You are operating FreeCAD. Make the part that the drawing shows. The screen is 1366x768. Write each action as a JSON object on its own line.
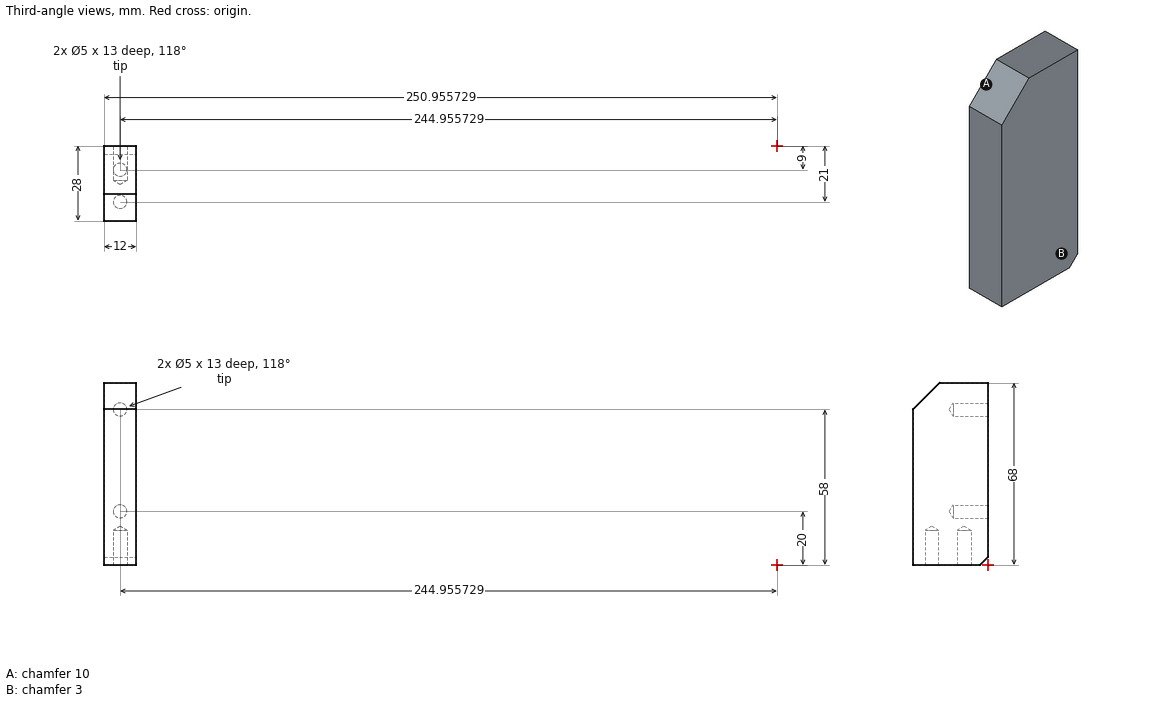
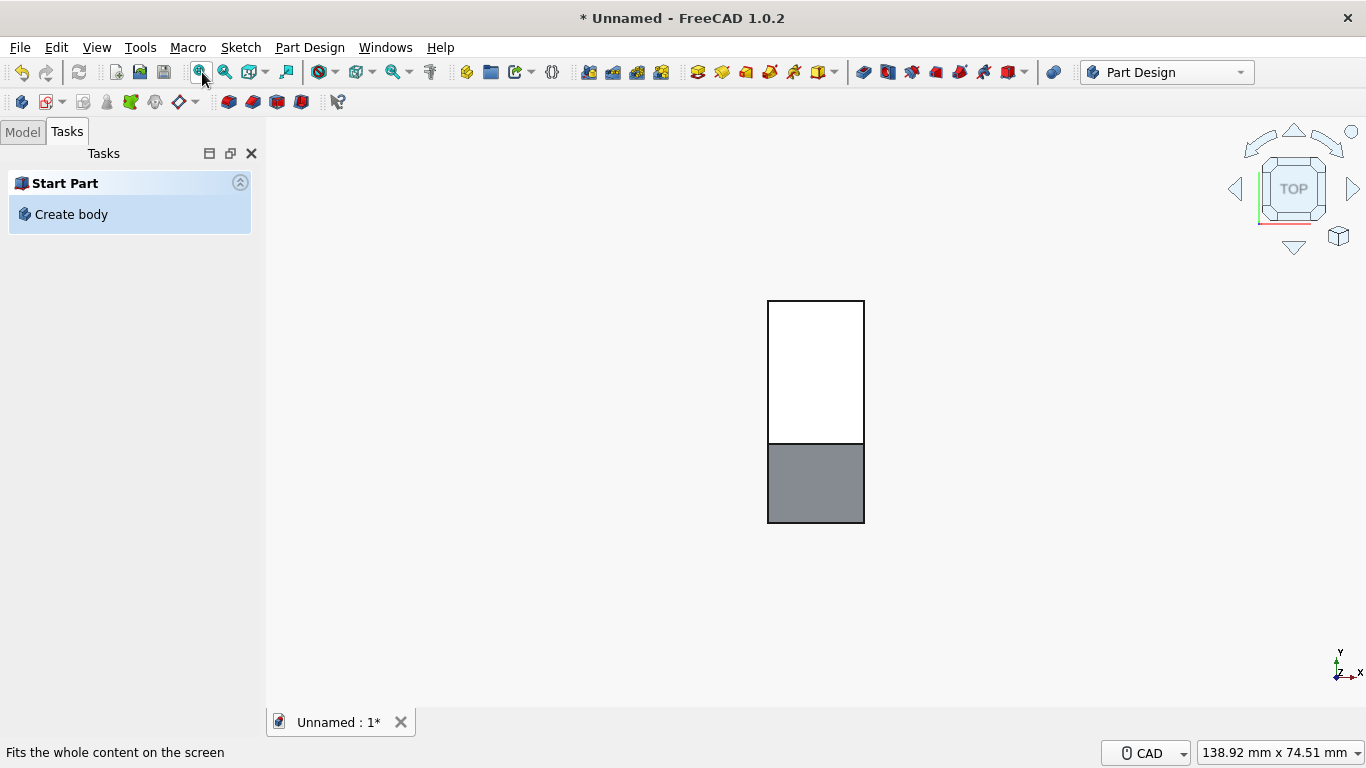
{"action": "key", "text": "1"}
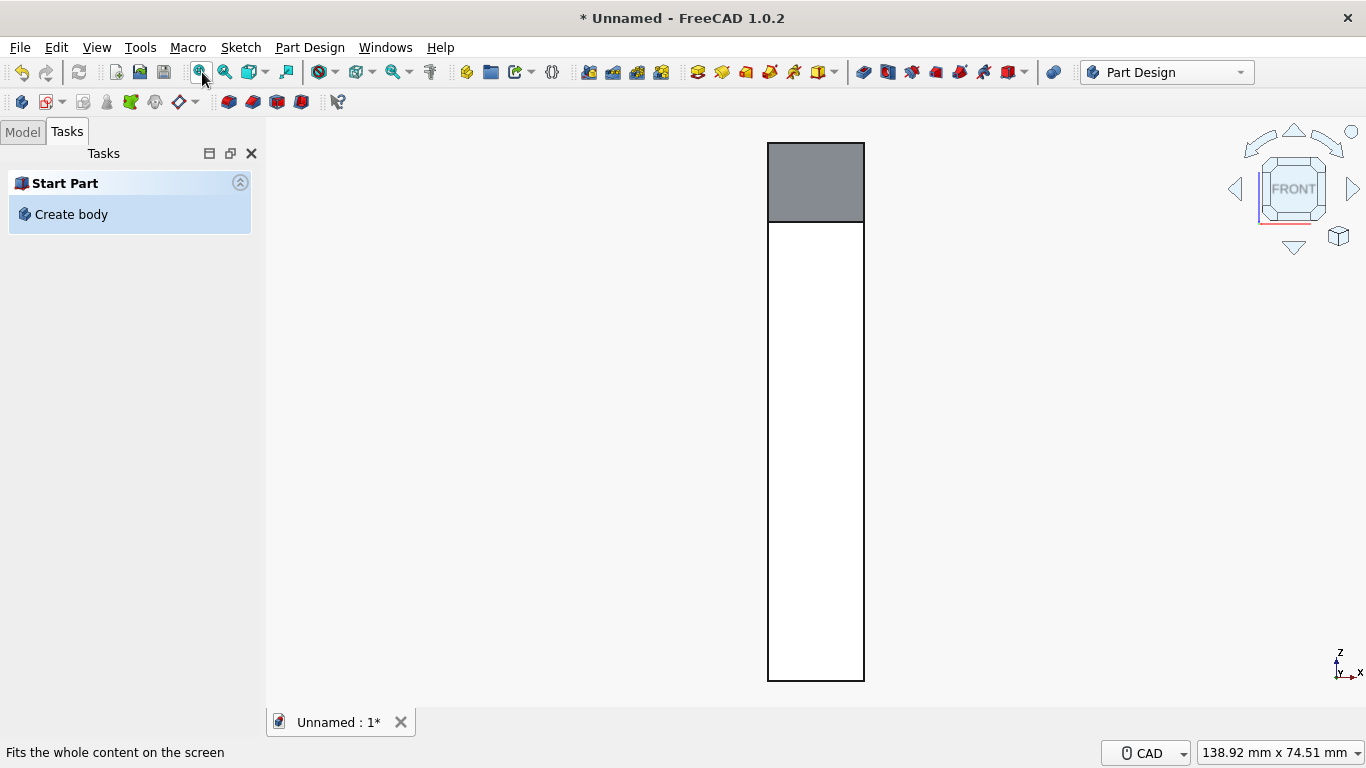
{"action": "key", "text": "3"}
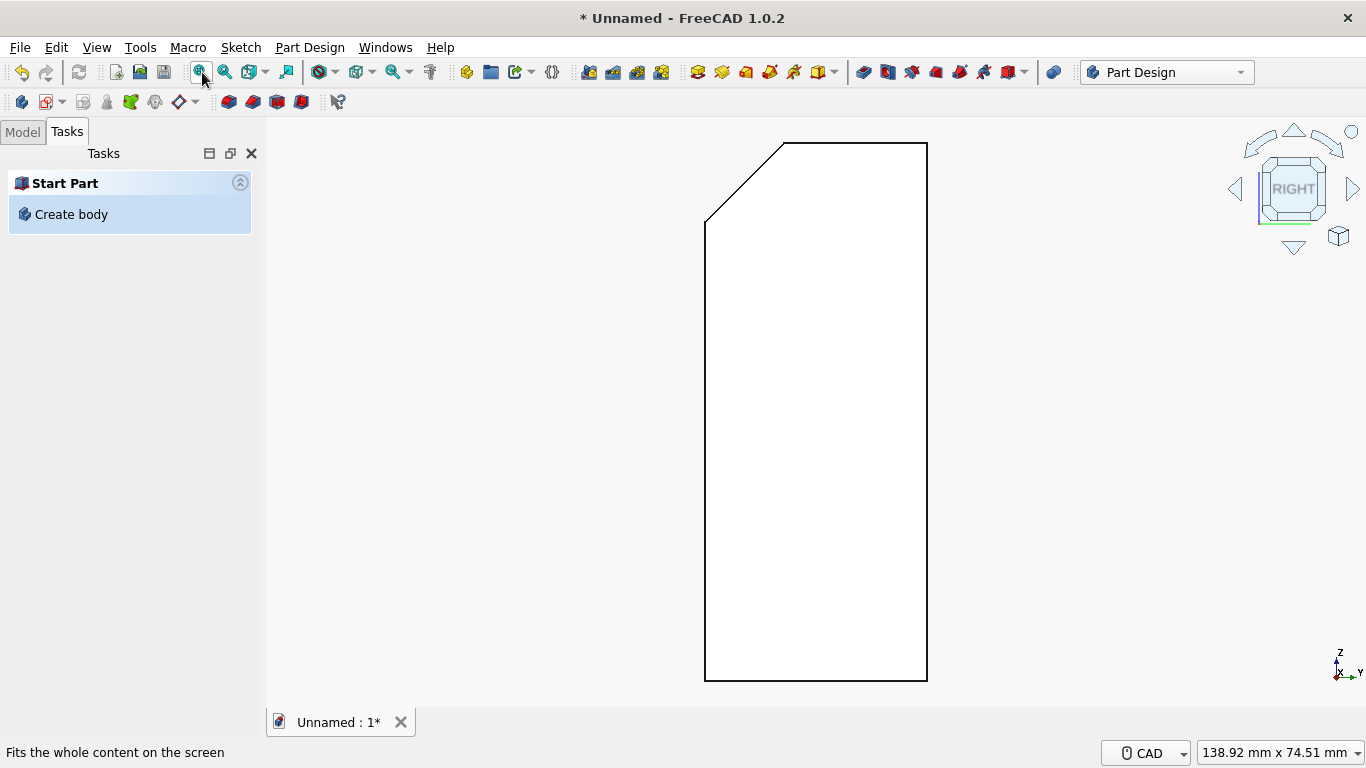
{"action": "key", "text": "5"}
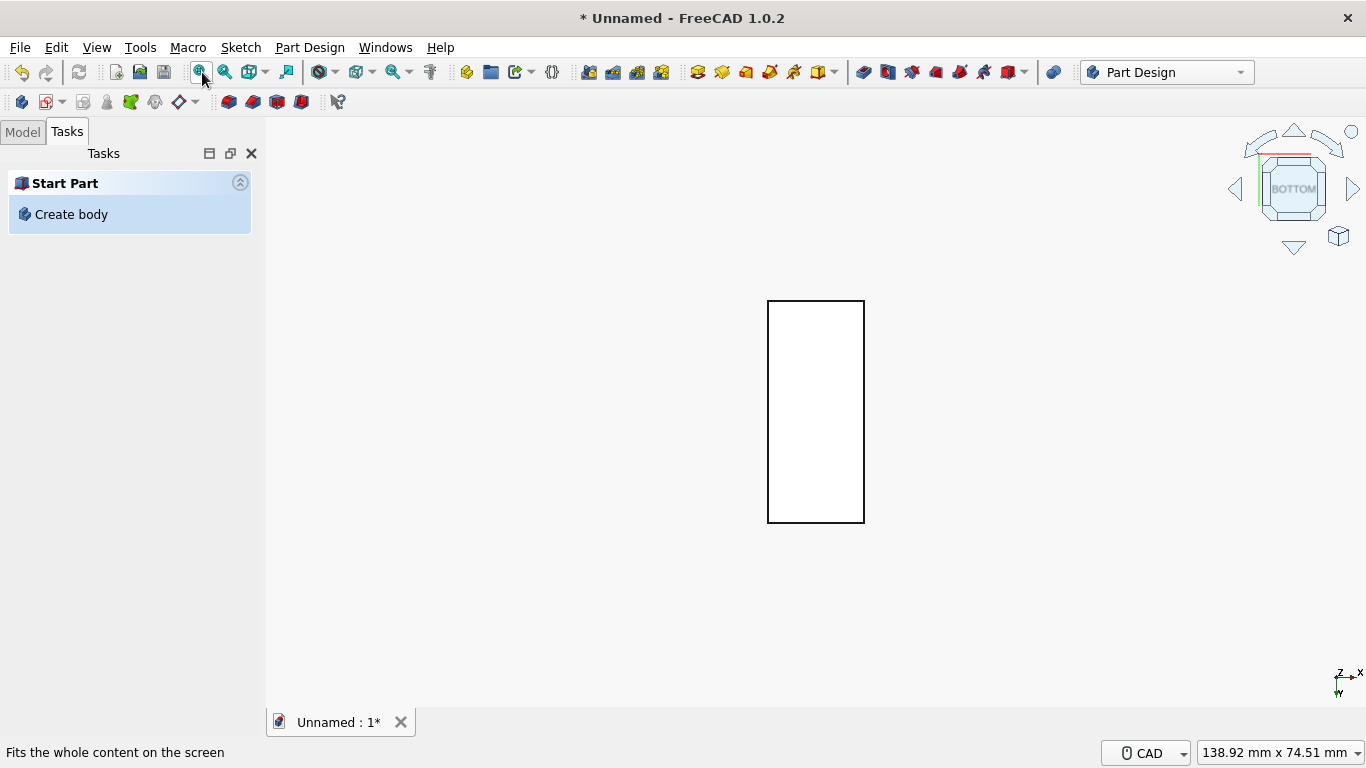
{"action": "left_click", "coordinate": [202, 72]}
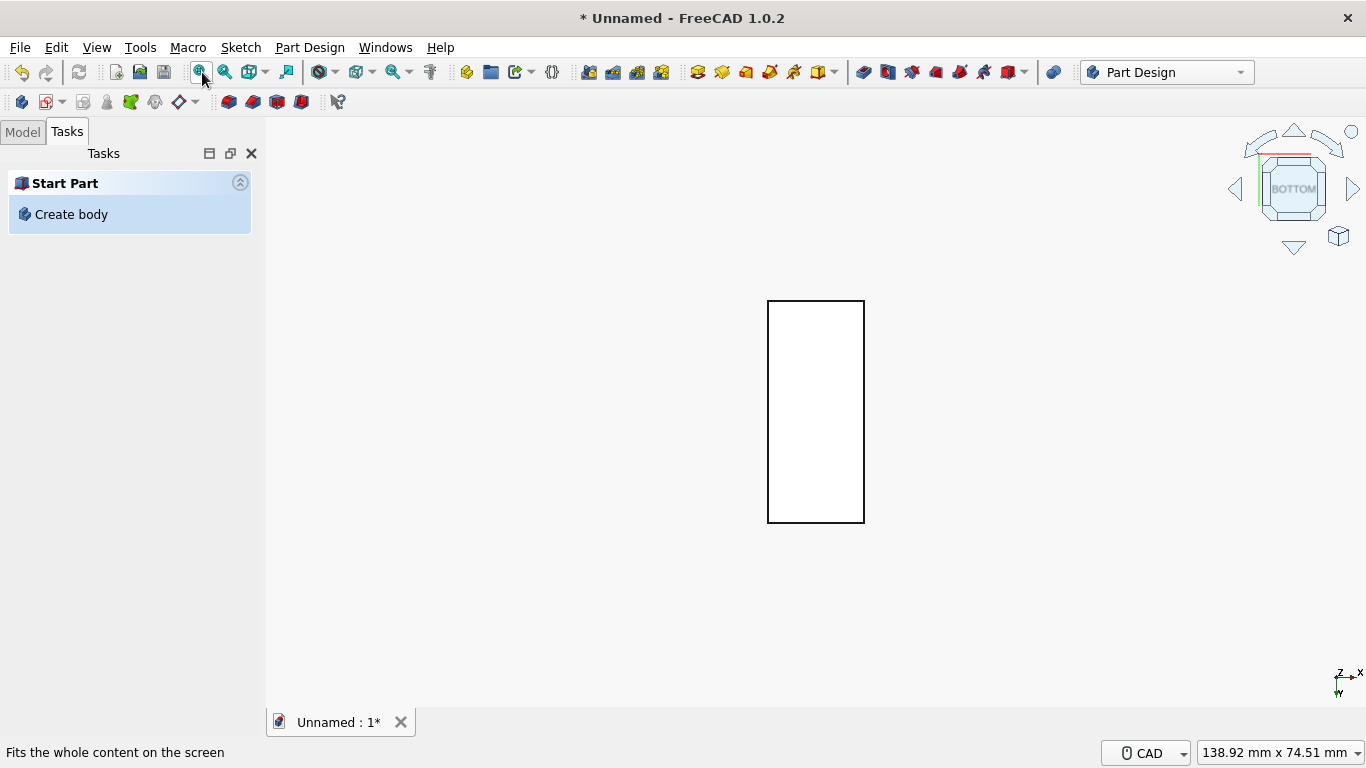
{"action": "left_click", "coordinate": [816, 522]}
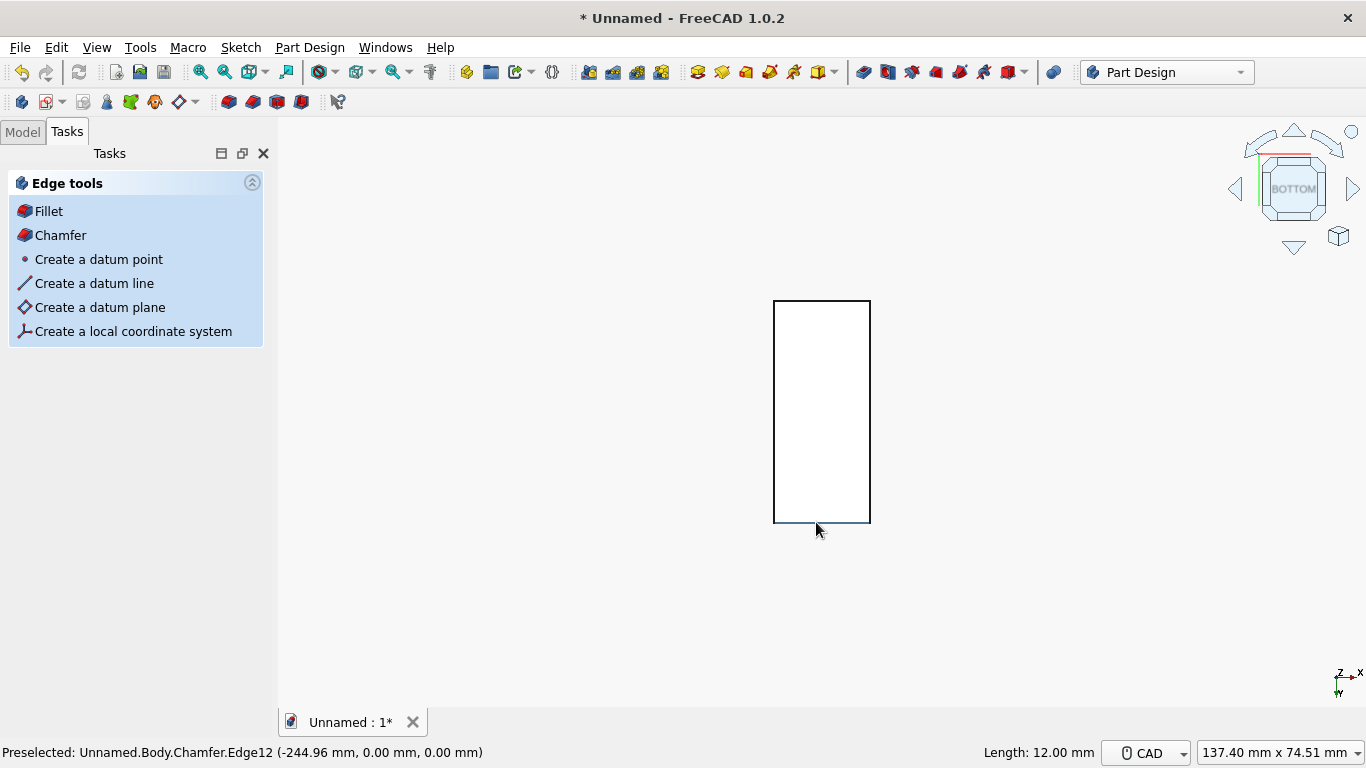
{"action": "left_click", "coordinate": [254, 102]}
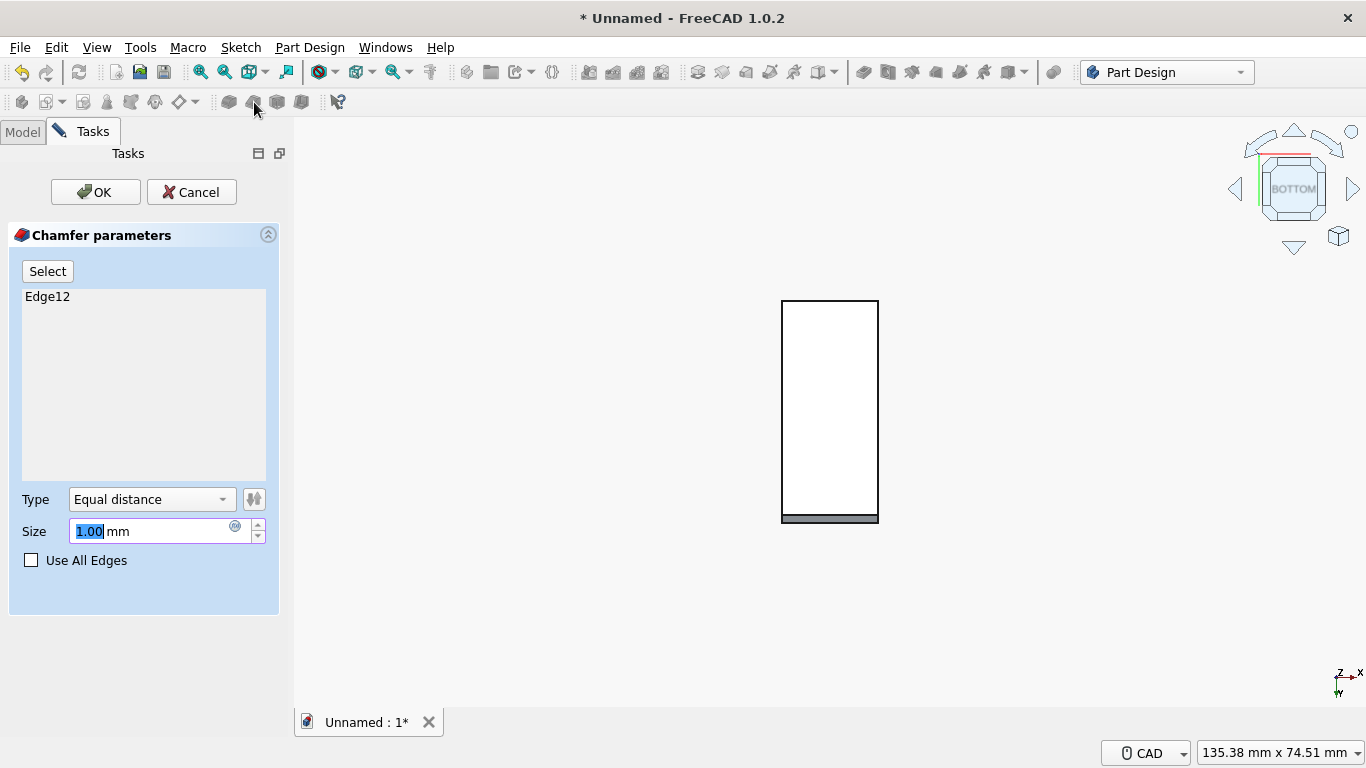
{"action": "type", "text": "3"}
{"action": "key", "text": "Tab"}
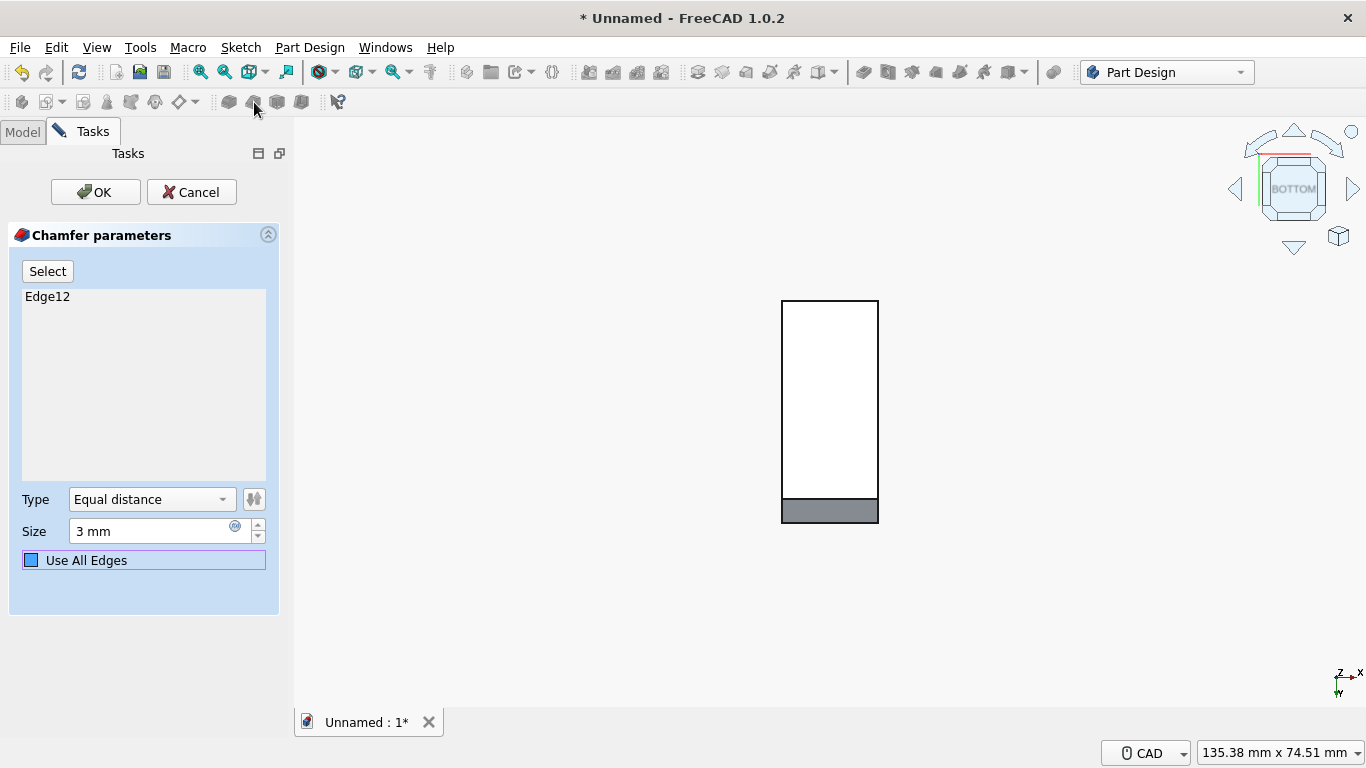
{"action": "left_click", "coordinate": [96, 192]}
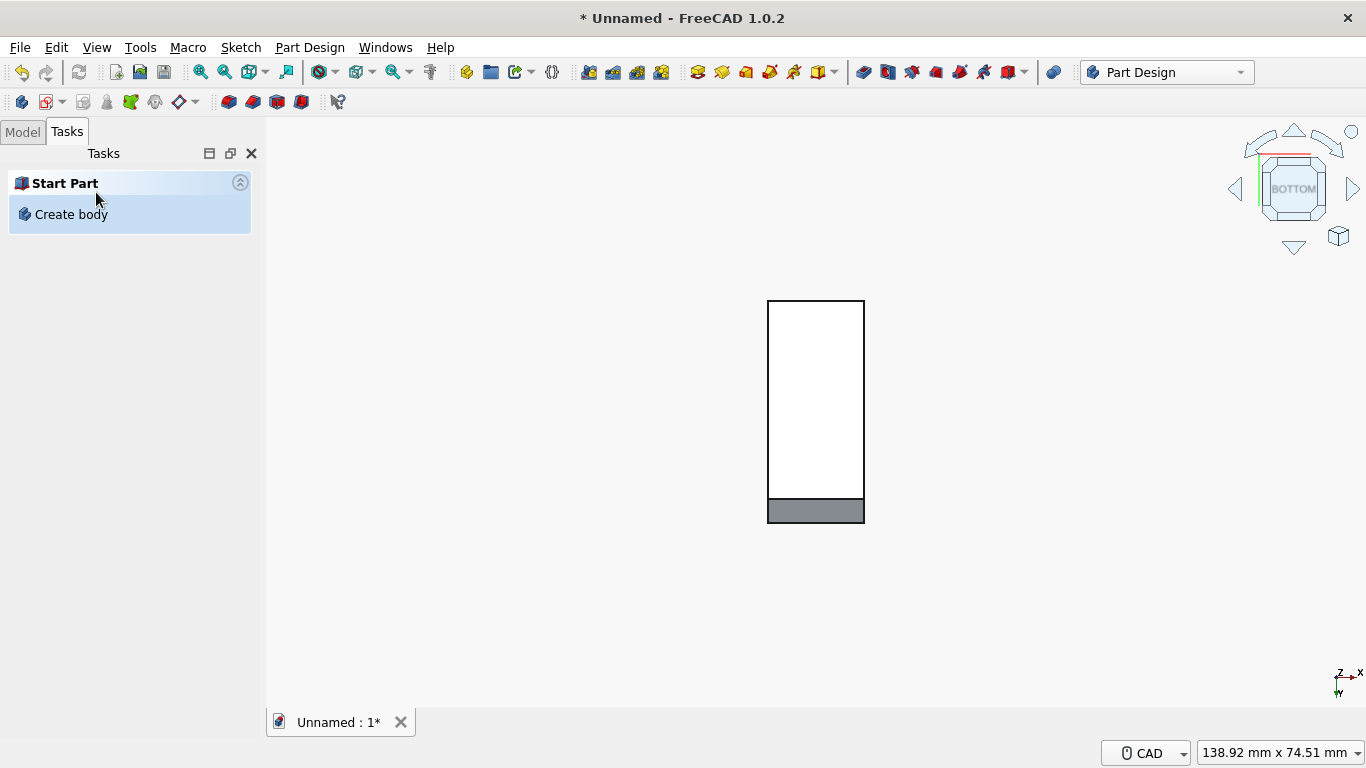
{"action": "left_click", "coordinate": [202, 72]}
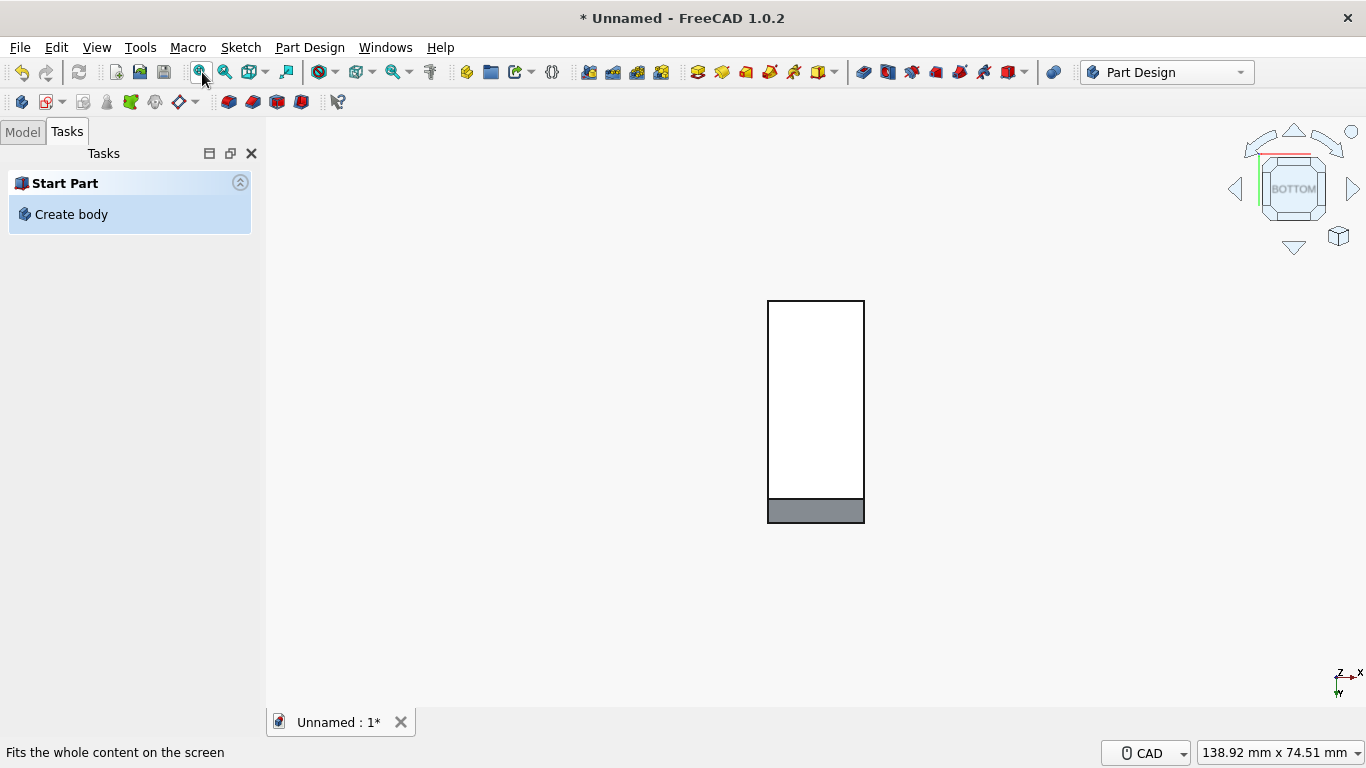
{"action": "left_click", "coordinate": [46, 102]}